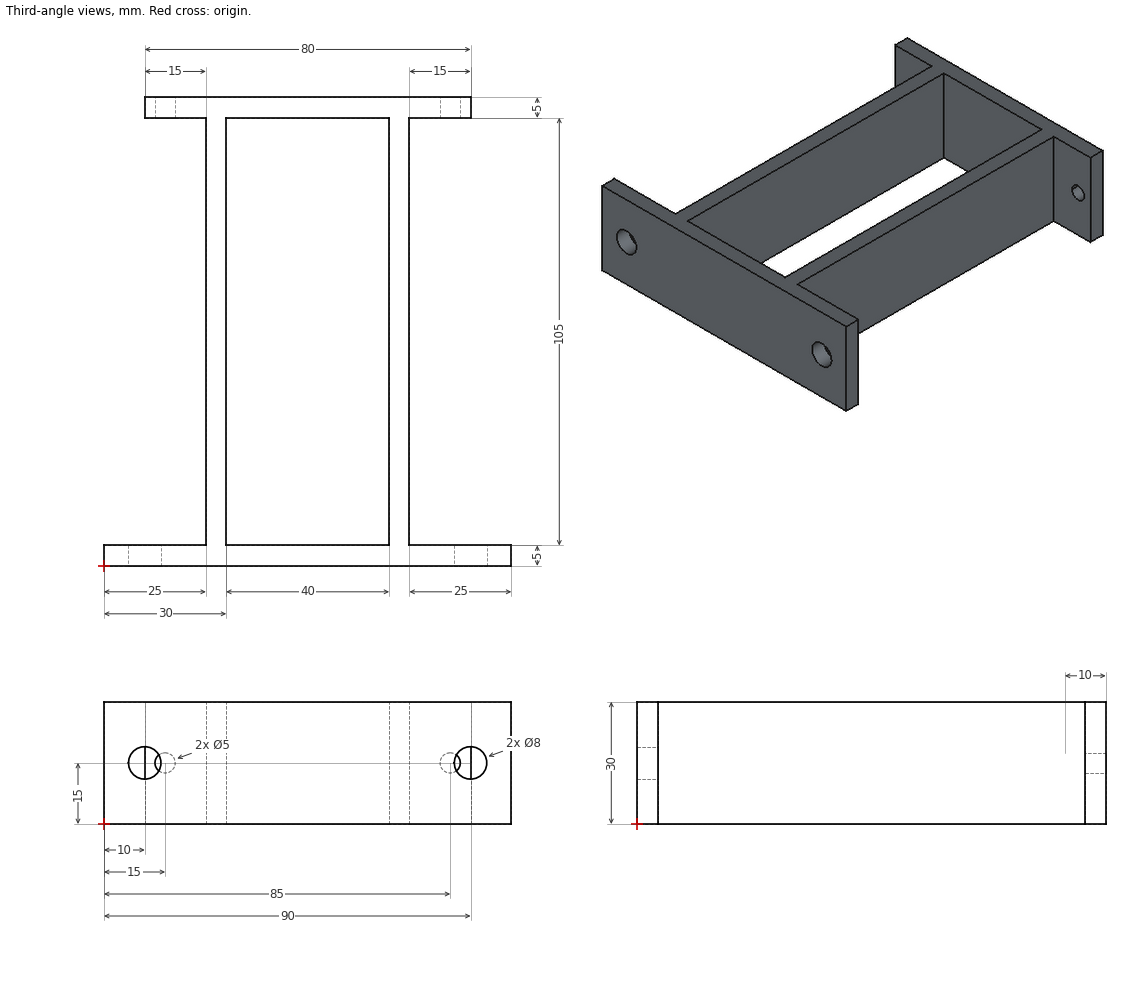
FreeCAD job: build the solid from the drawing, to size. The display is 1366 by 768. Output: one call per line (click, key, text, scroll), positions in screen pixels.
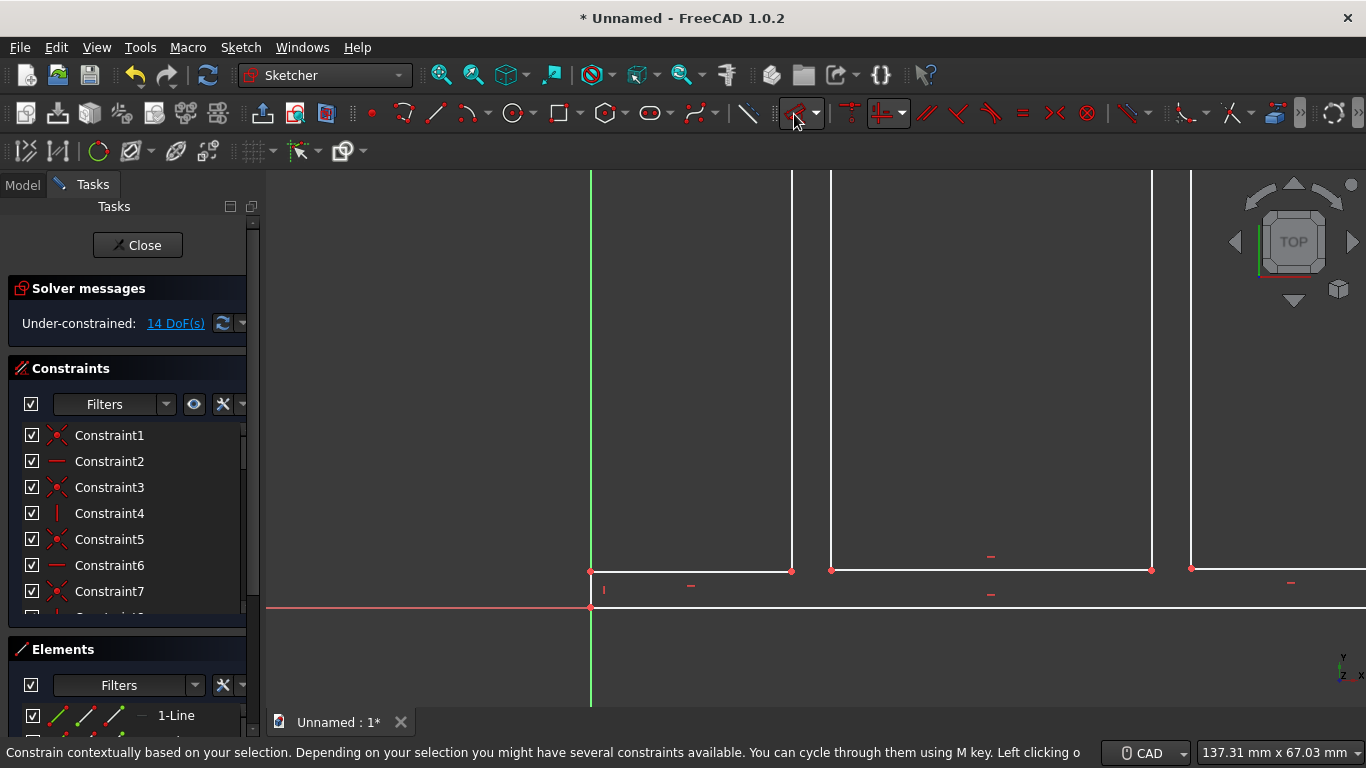
scroll(606, 608, down, 5)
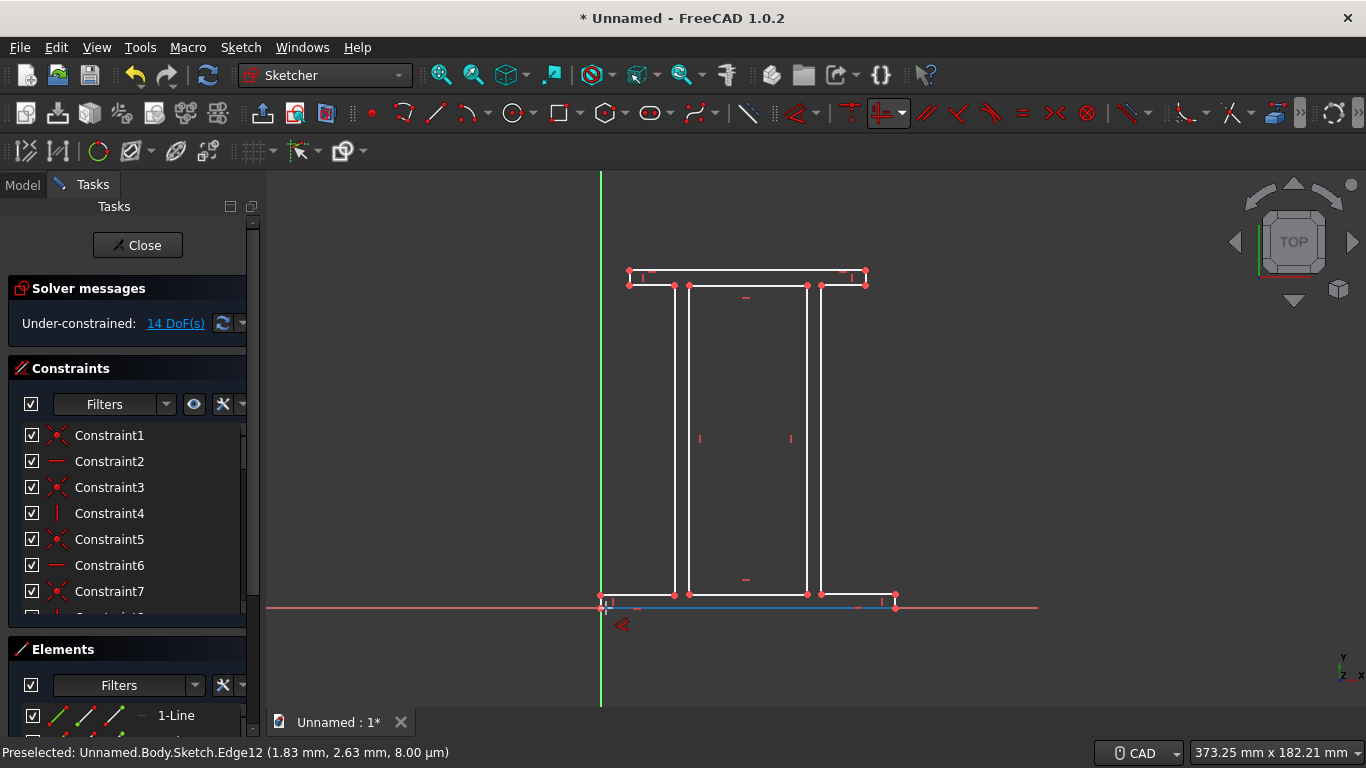
scroll(895, 604, up, 6)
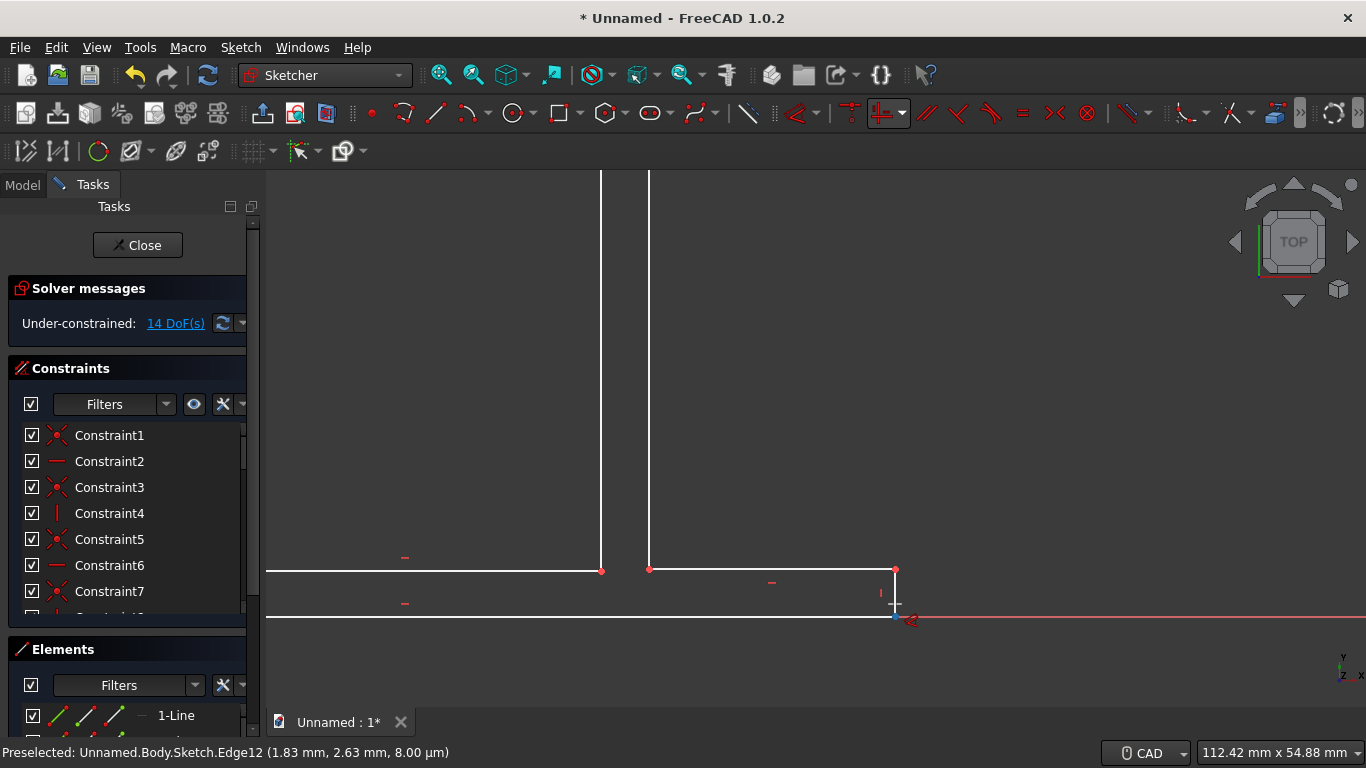
click(895, 602)
click(929, 593)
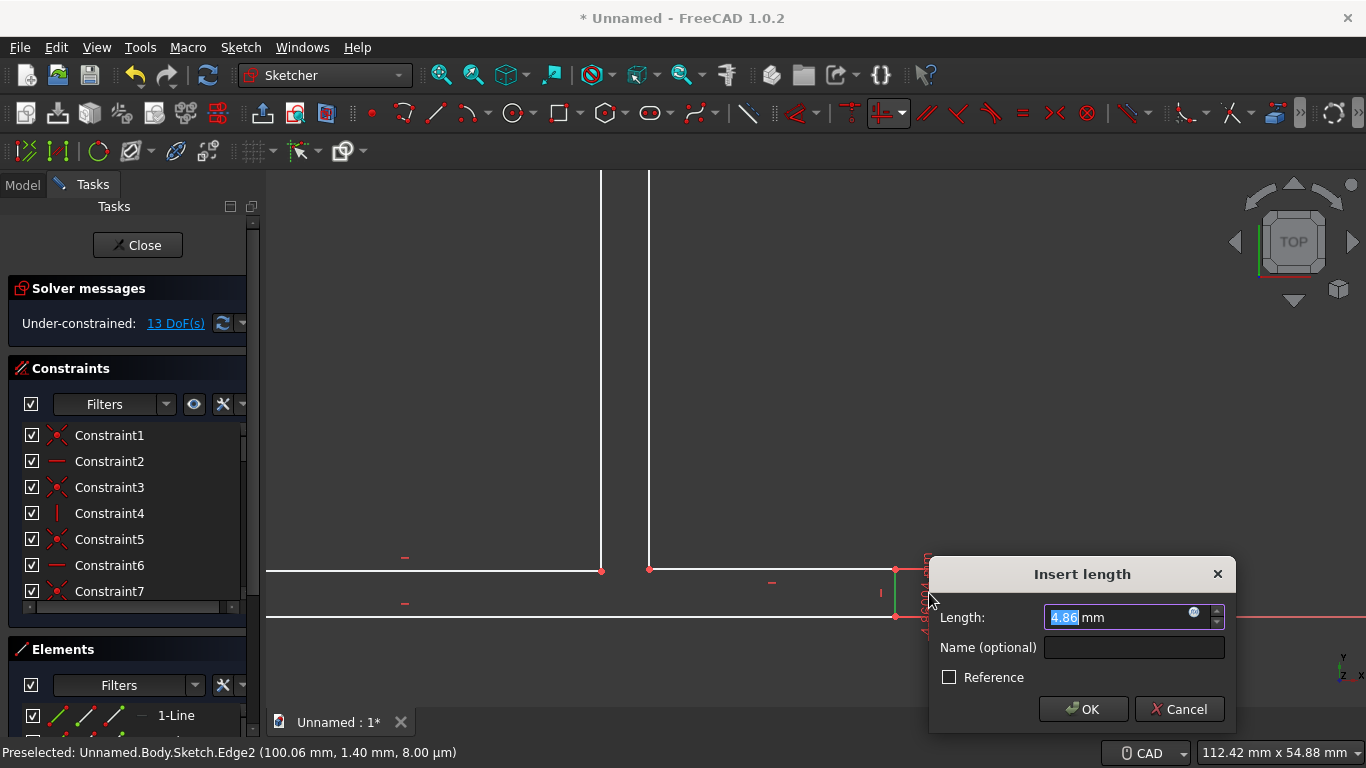
text(5)
key(Return)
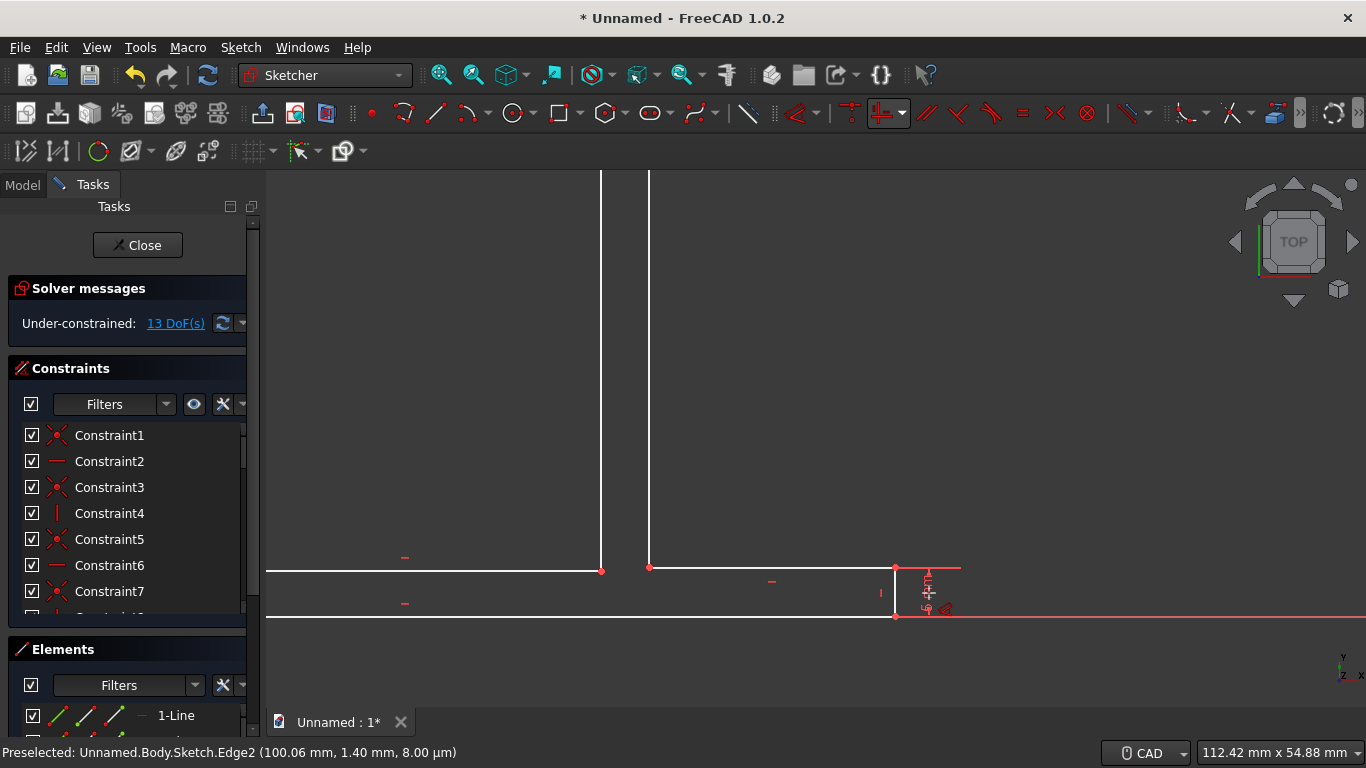
scroll(895, 604, down, 6)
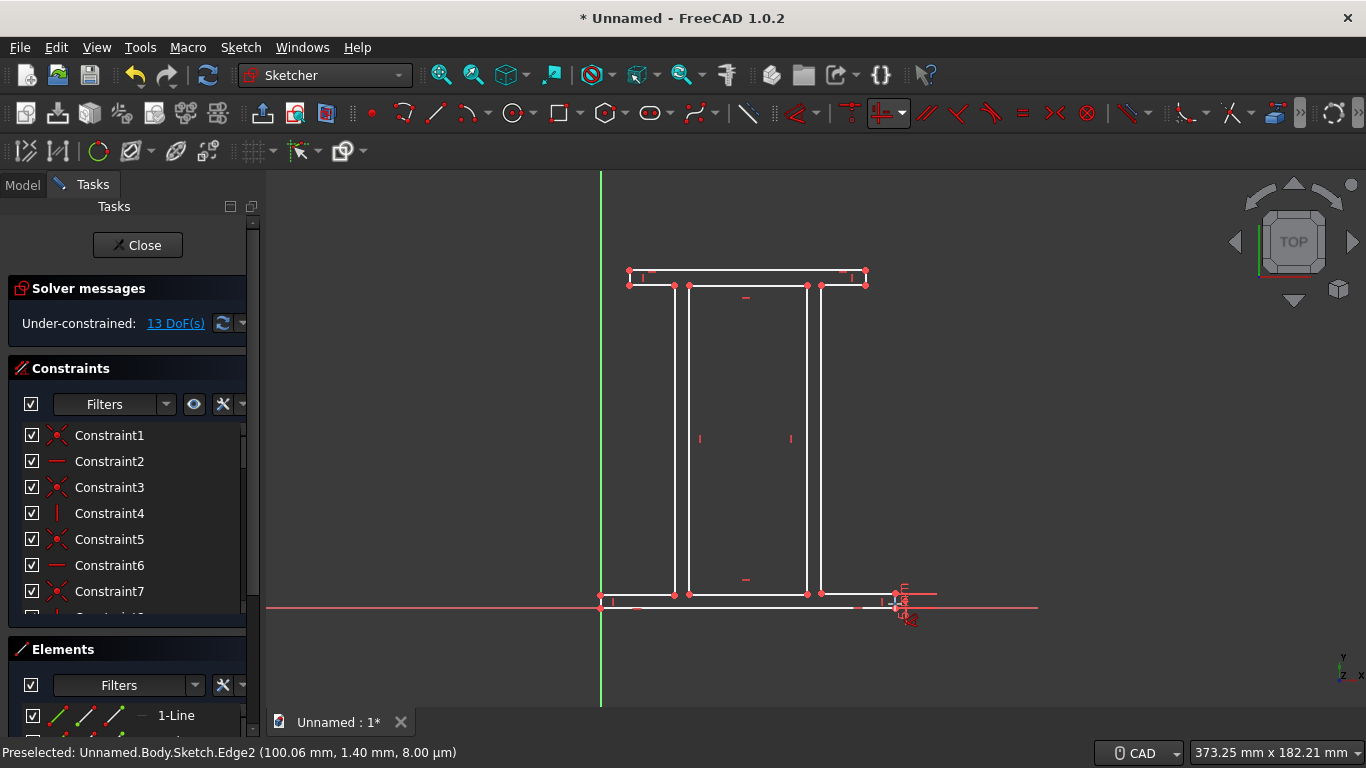
scroll(866, 281, up, 6)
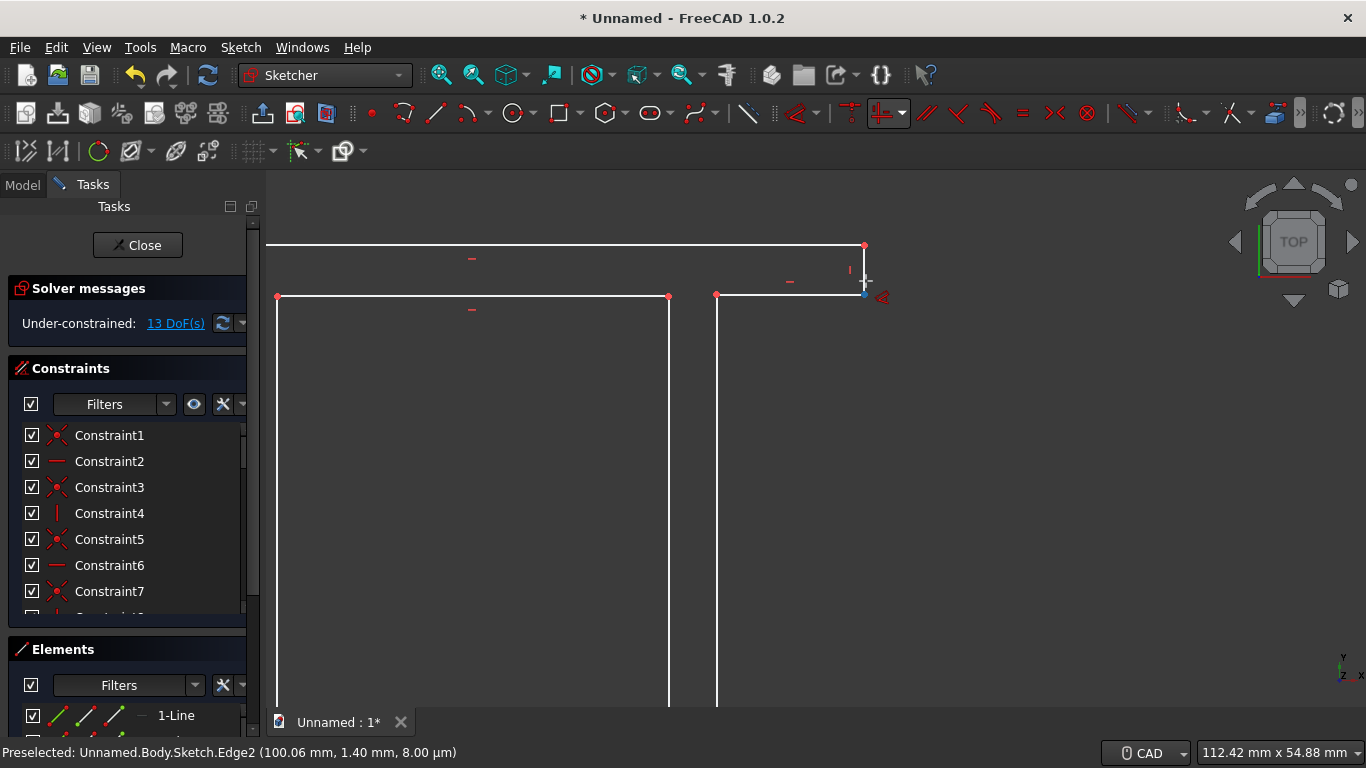
click(864, 280)
click(898, 270)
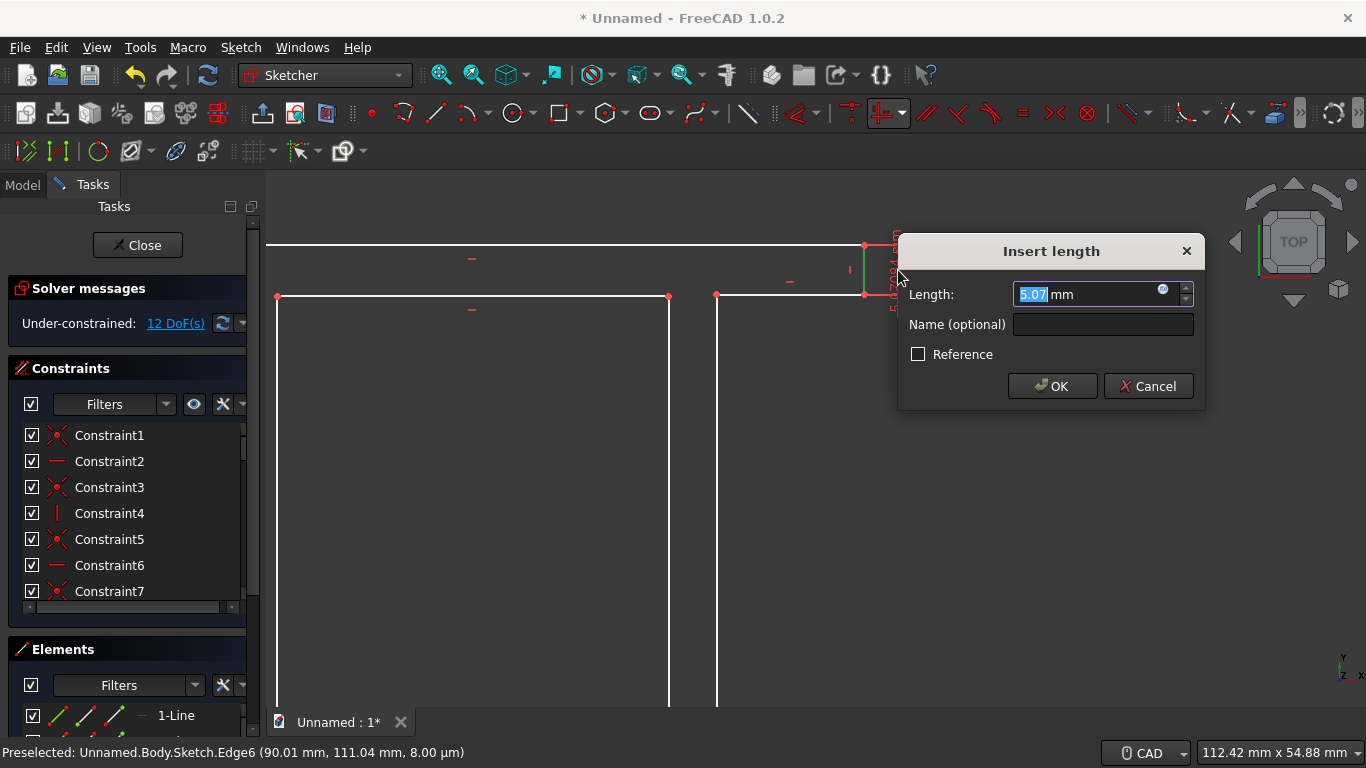
text(5)
key(Return)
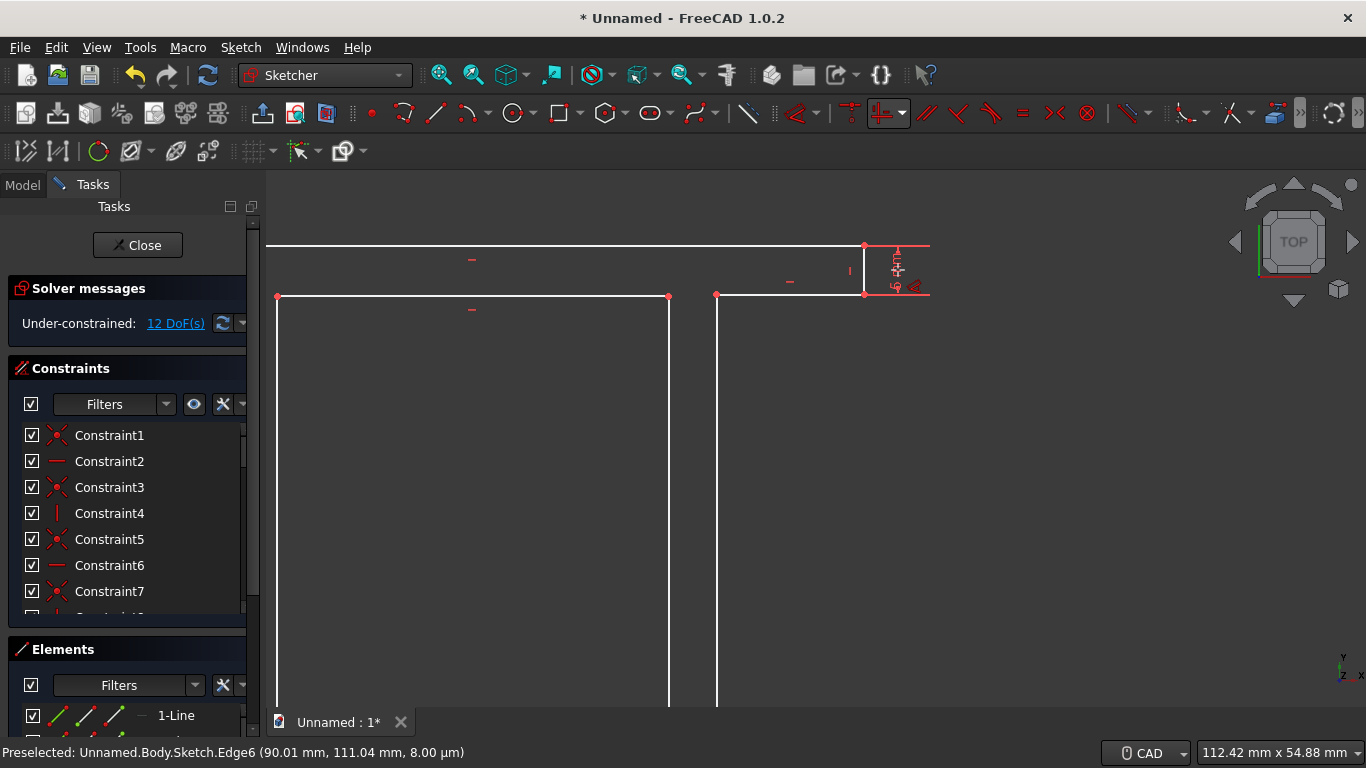
scroll(866, 281, down, 6)